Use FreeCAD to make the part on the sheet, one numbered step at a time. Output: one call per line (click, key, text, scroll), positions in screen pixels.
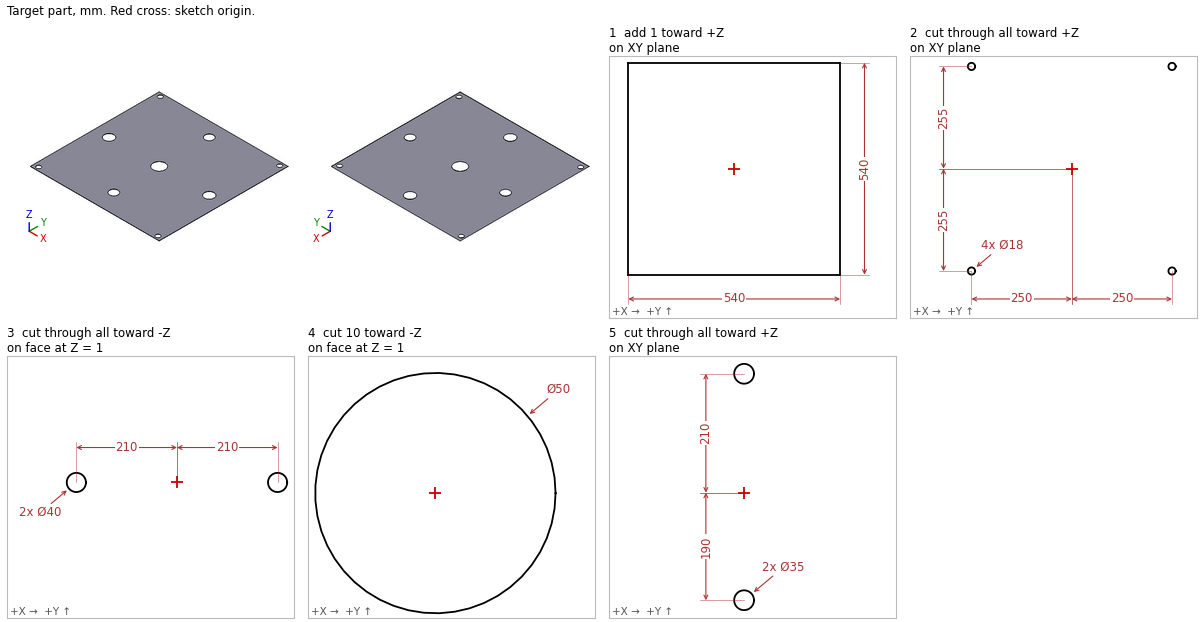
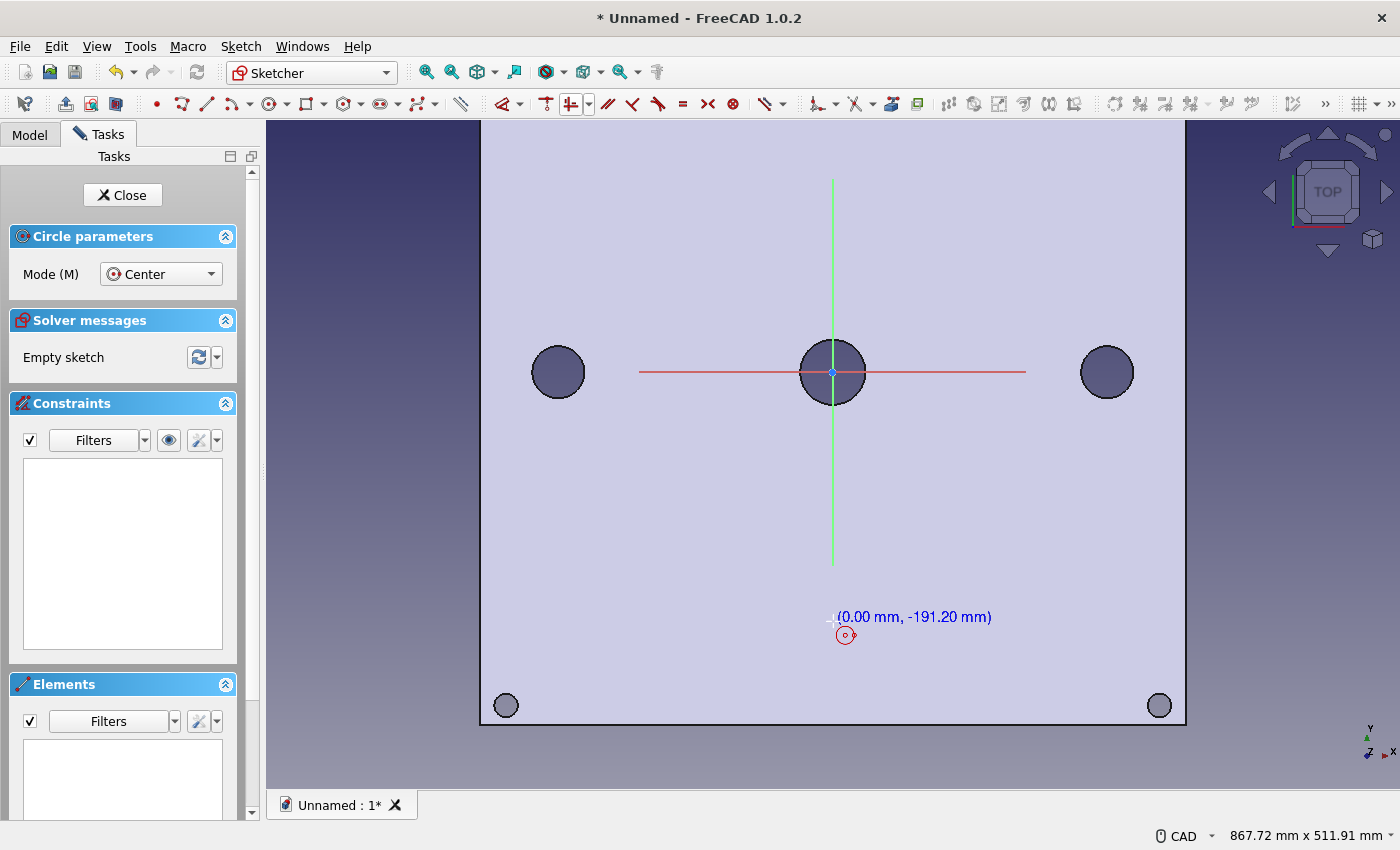
click(833, 621)
move(849, 604)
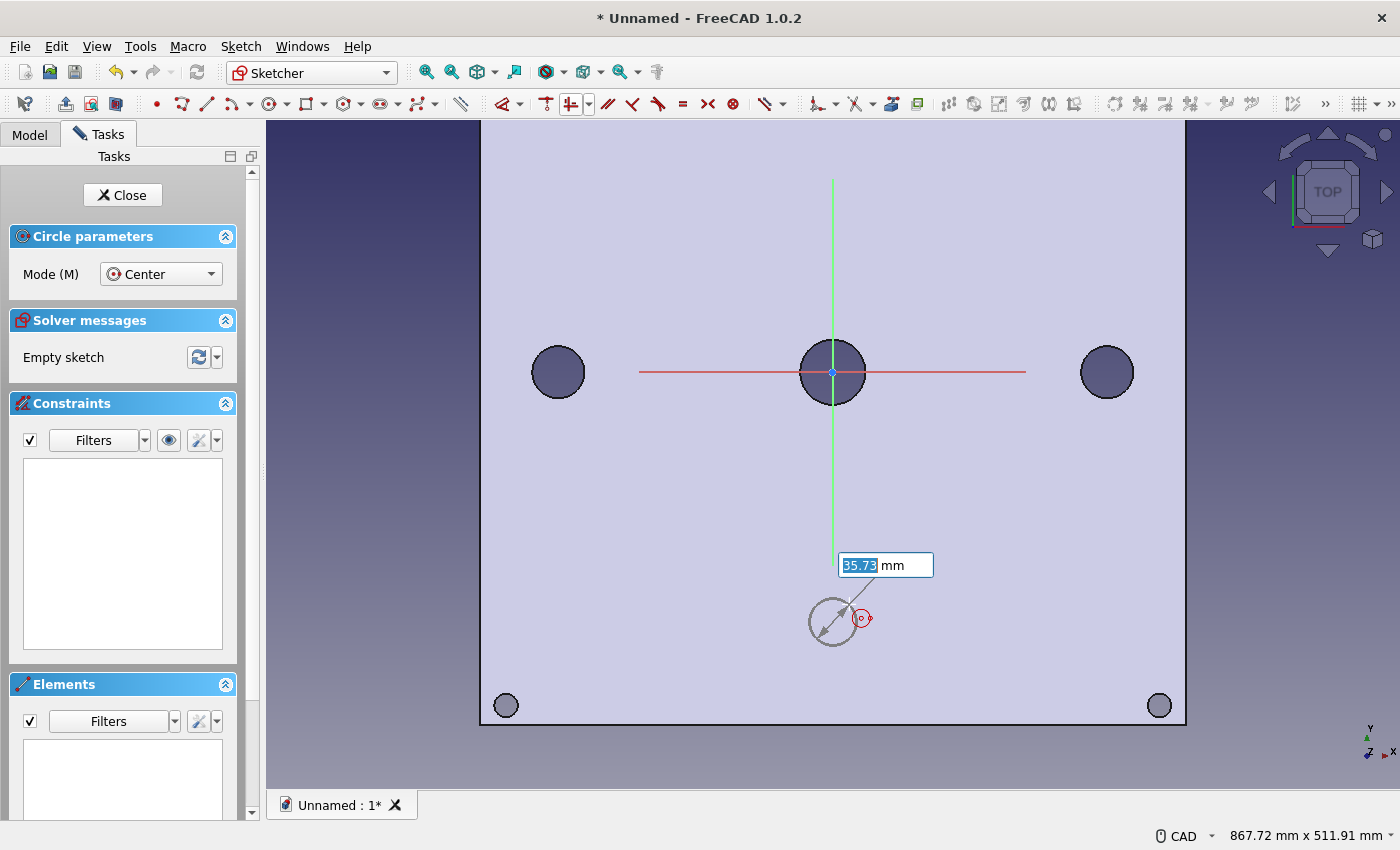
text(35)
key(Return)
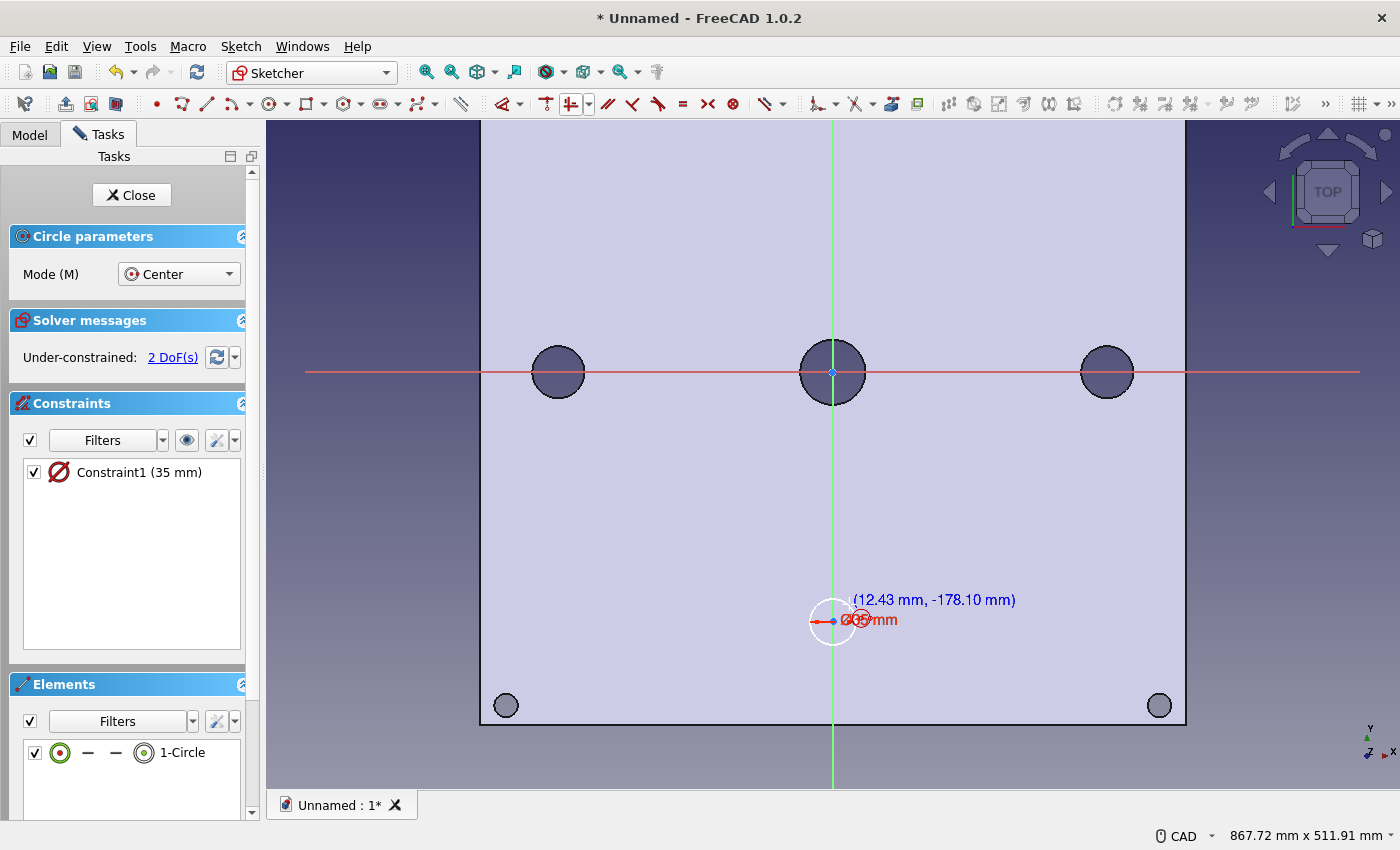
scroll(456, 761, down, 1)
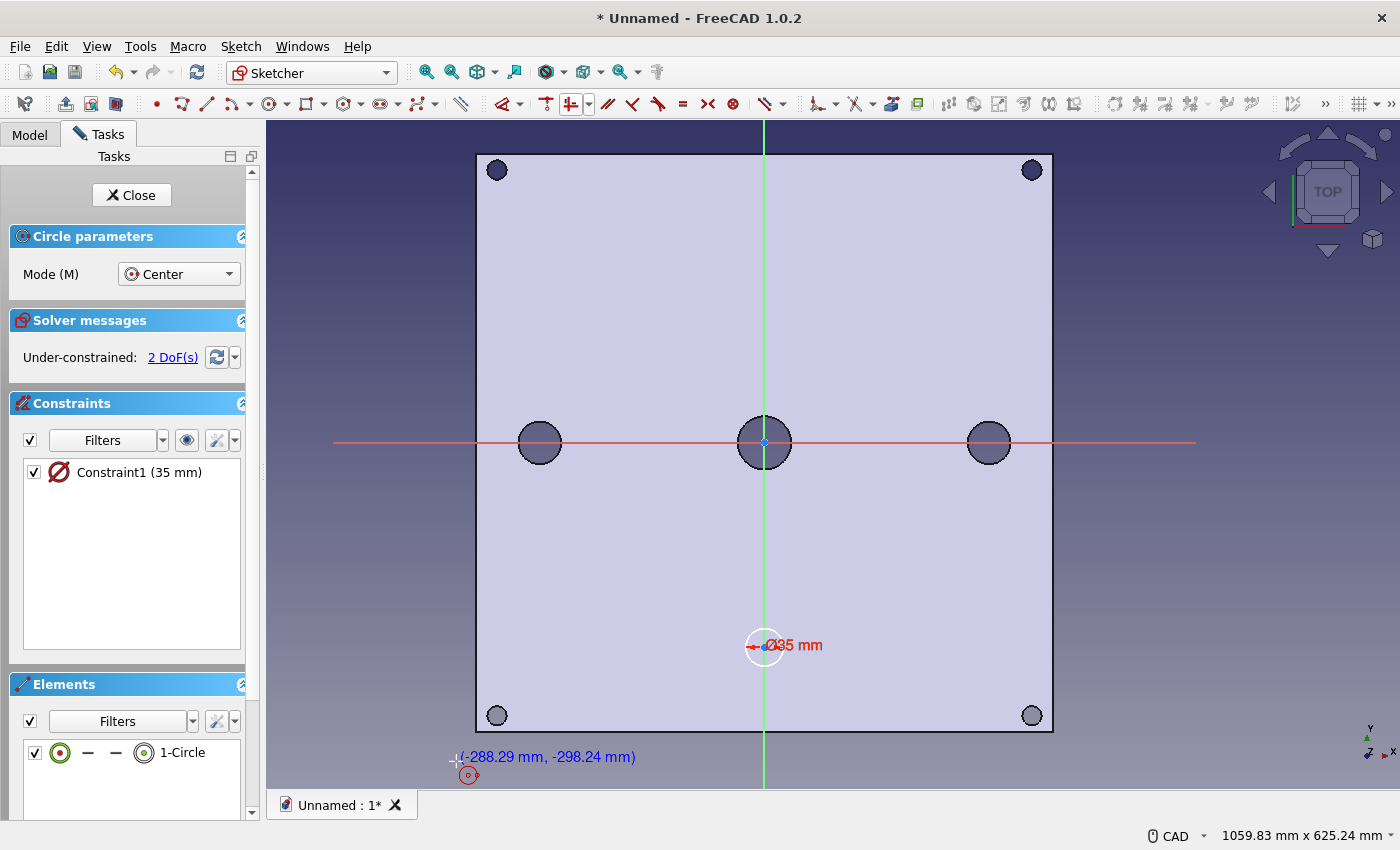
click(764, 218)
move(782, 212)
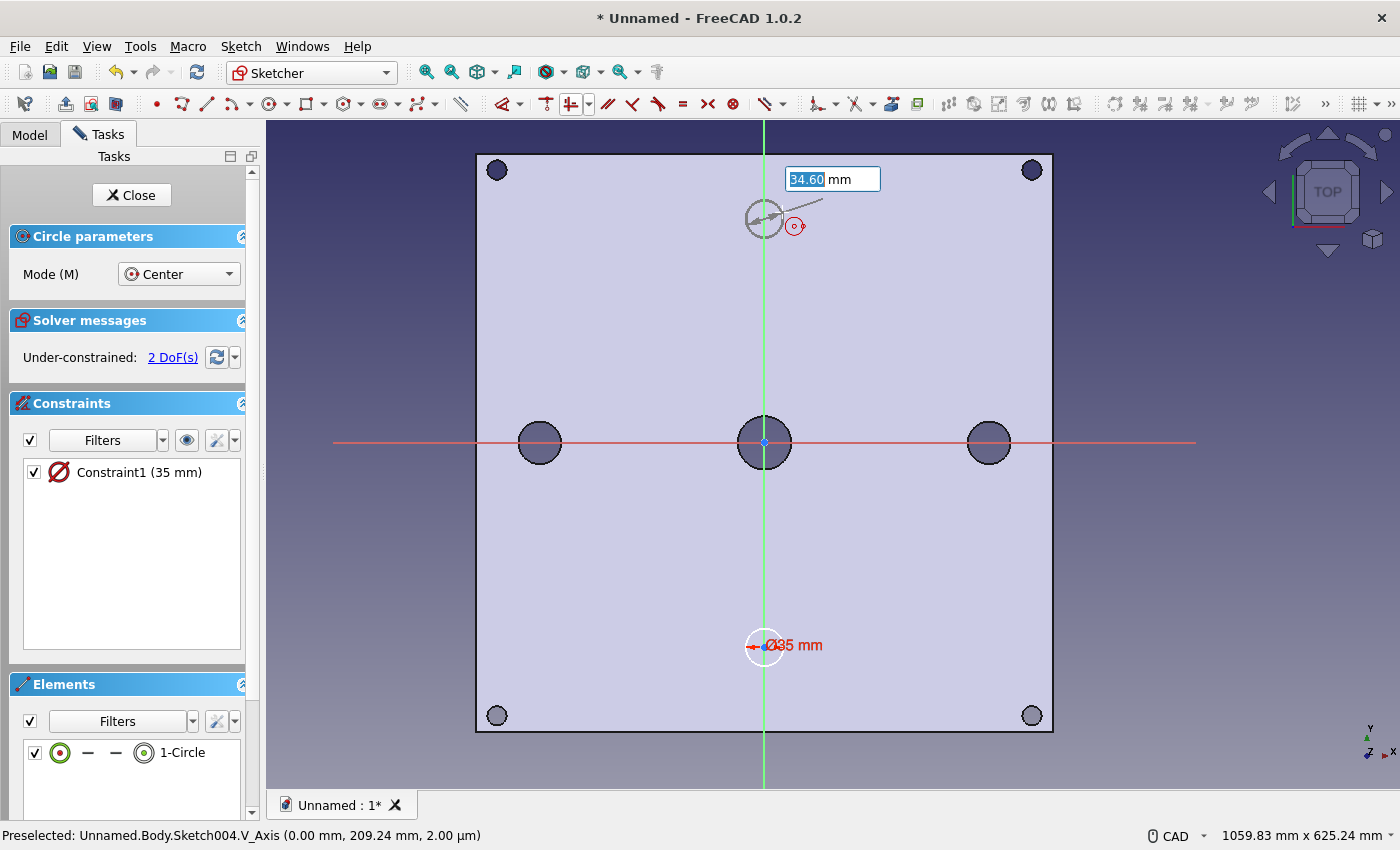
text(35)
key(Return)
key(Escape)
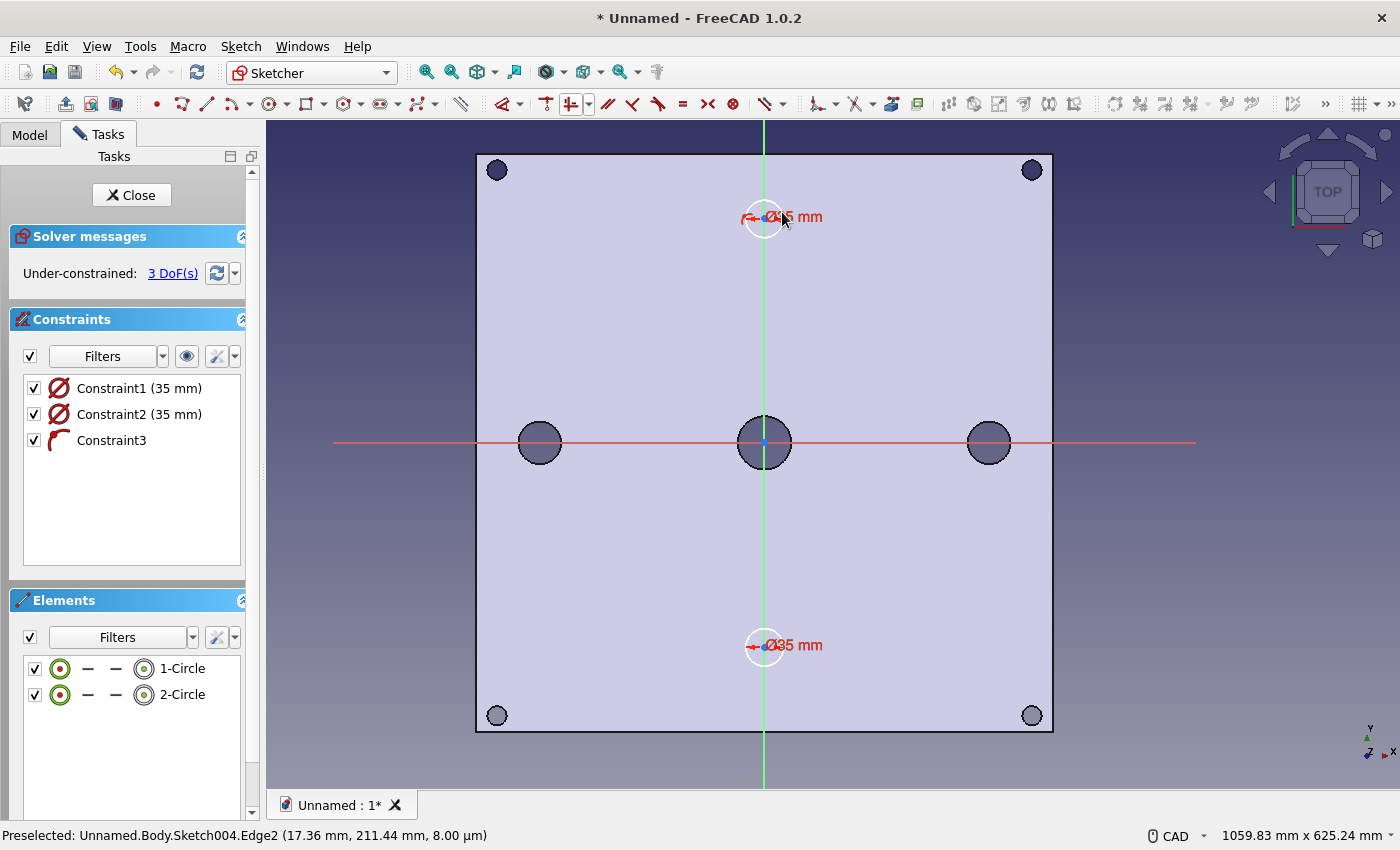
click(765, 647)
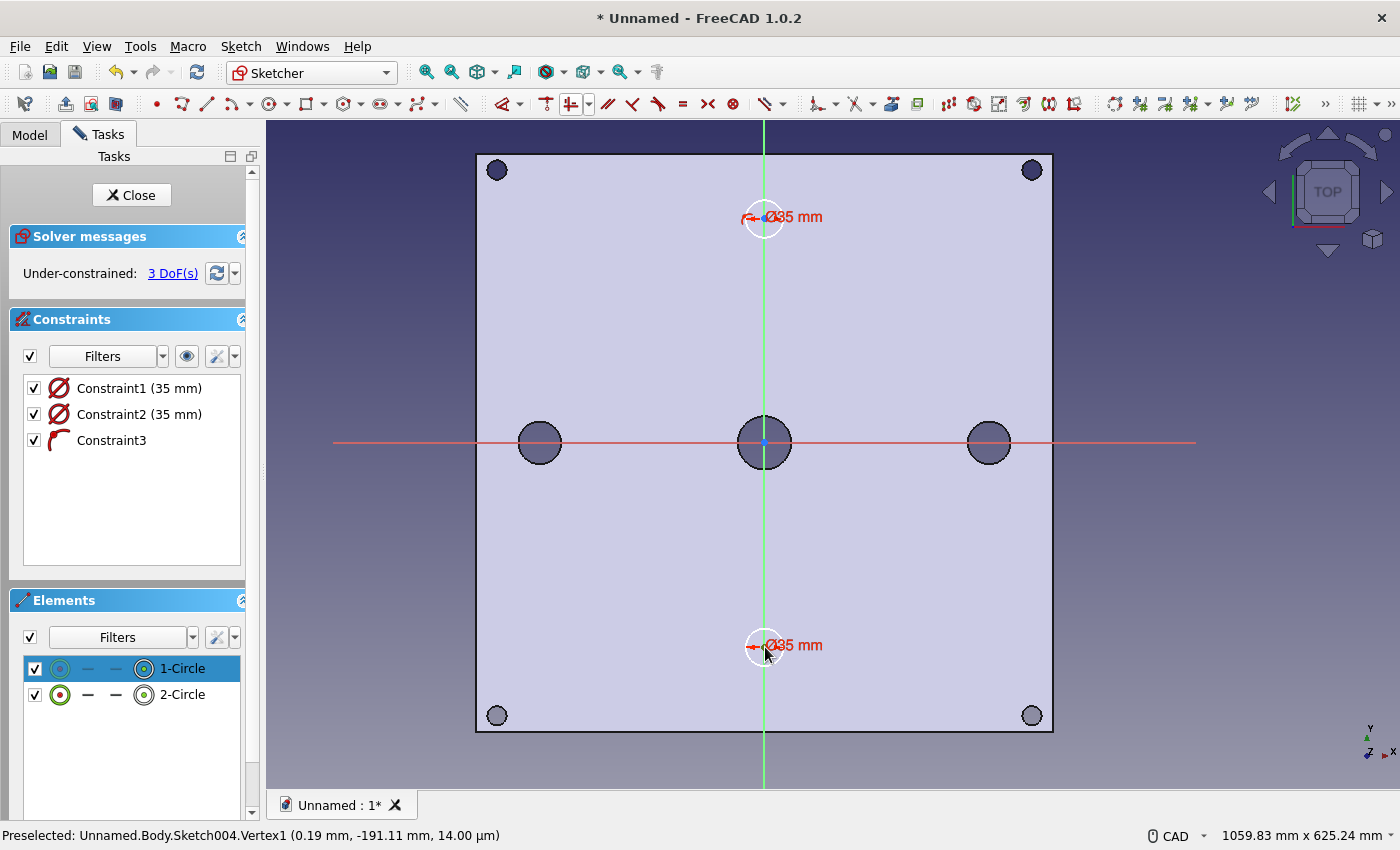
click(764, 717)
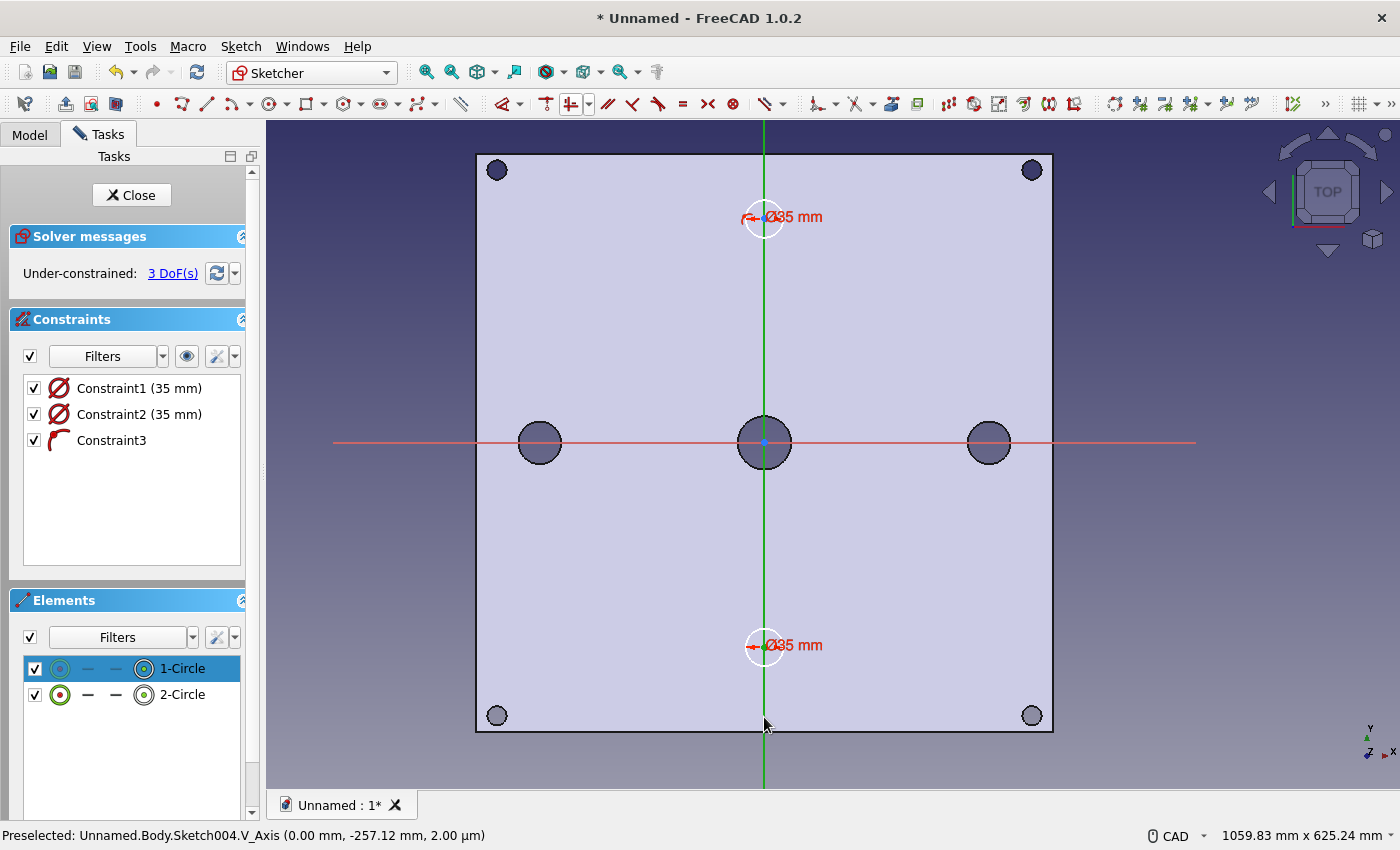
key(c)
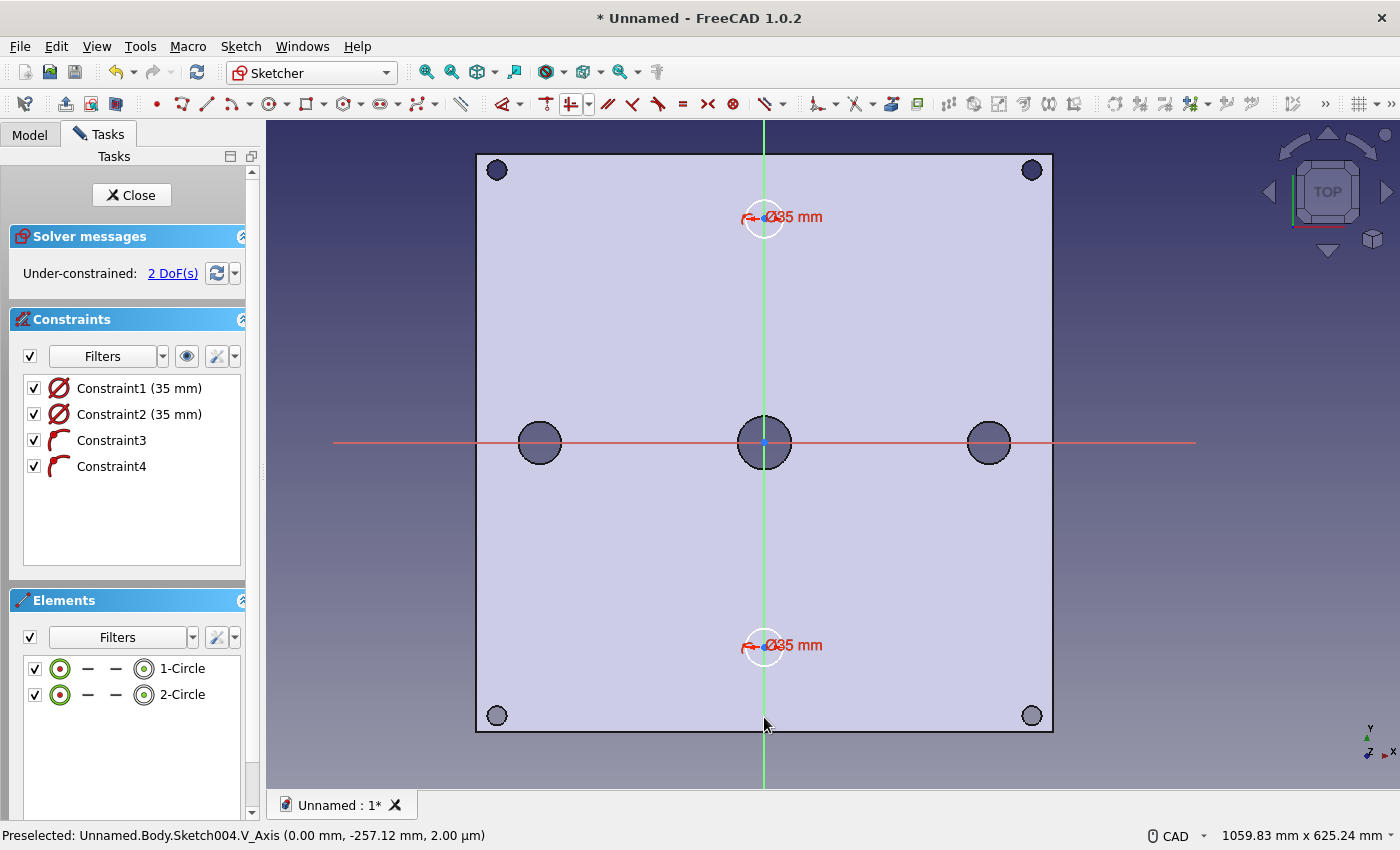
key(d)